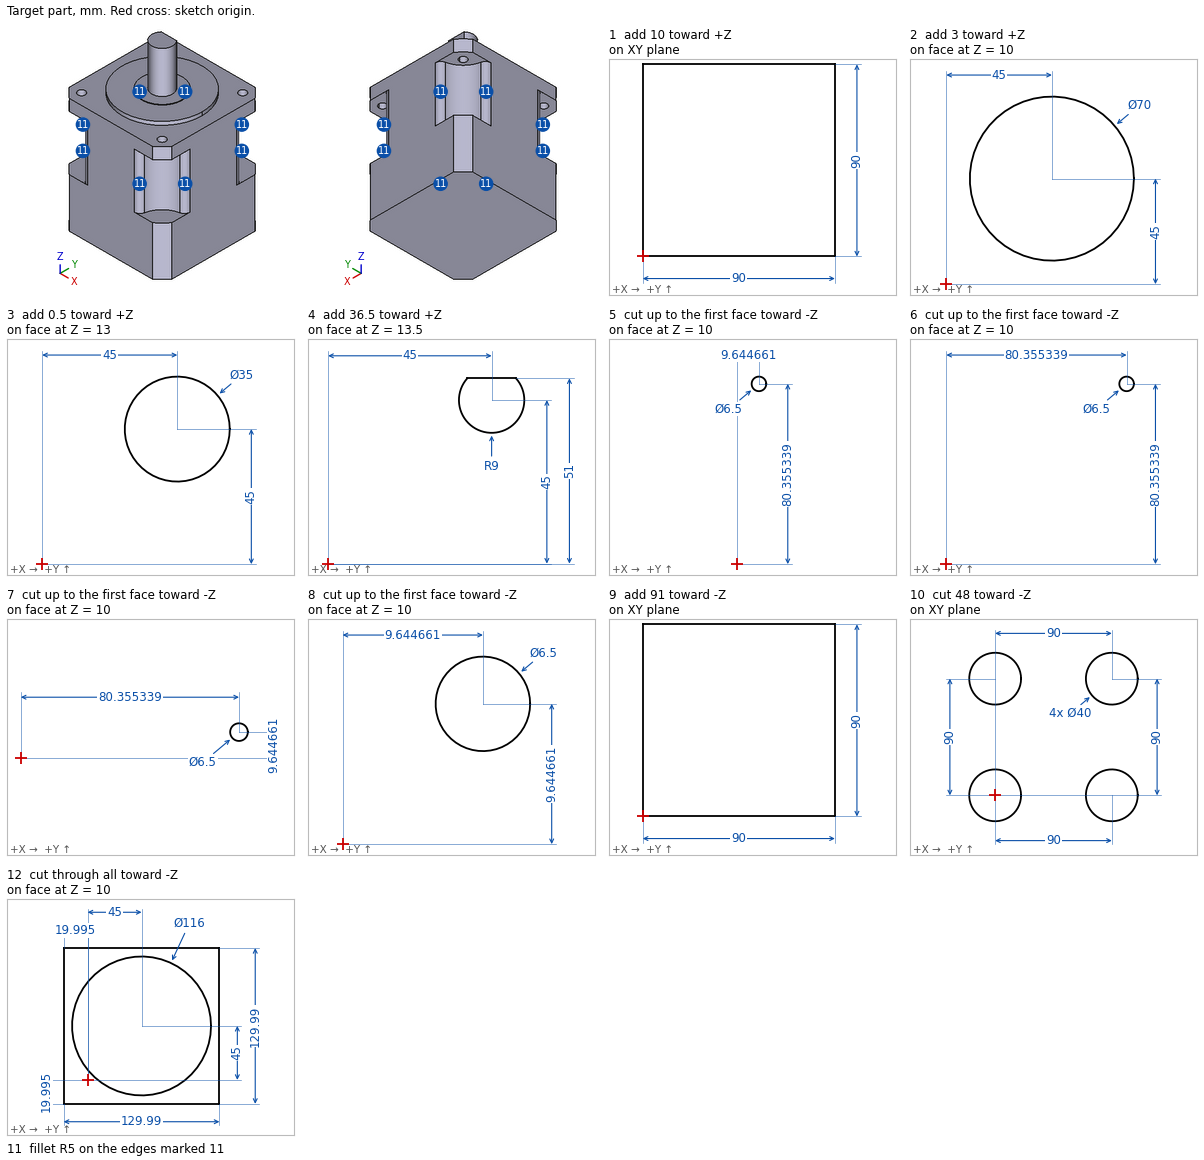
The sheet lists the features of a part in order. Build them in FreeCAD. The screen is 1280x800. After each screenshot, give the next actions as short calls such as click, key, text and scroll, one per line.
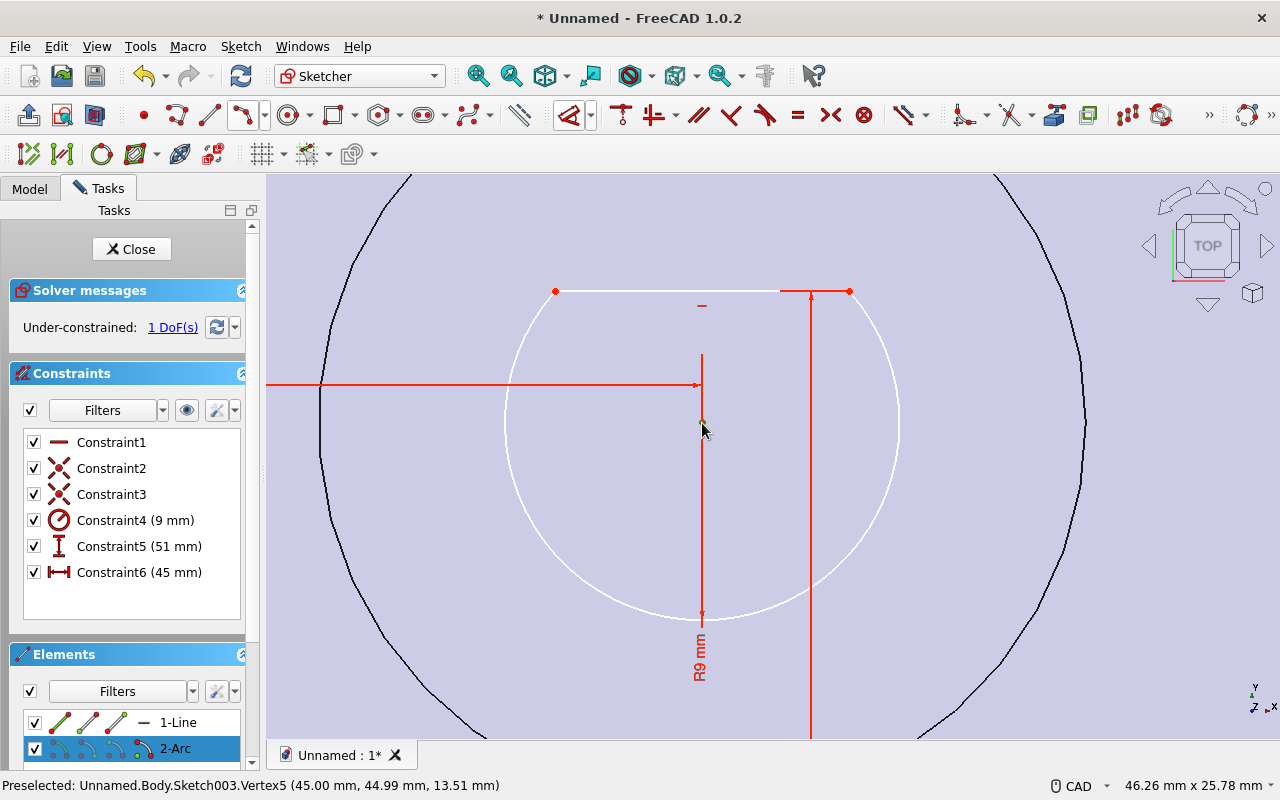
key(i)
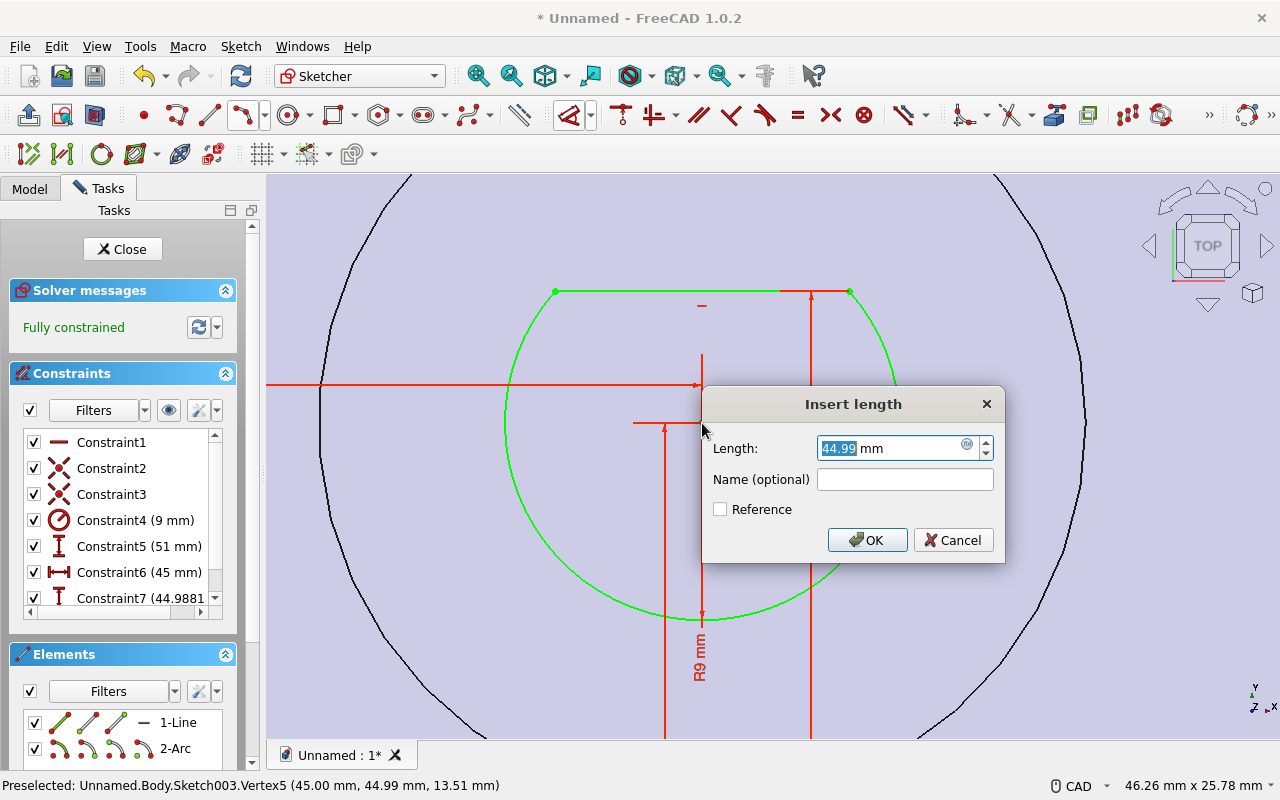
text(45)
key(Return)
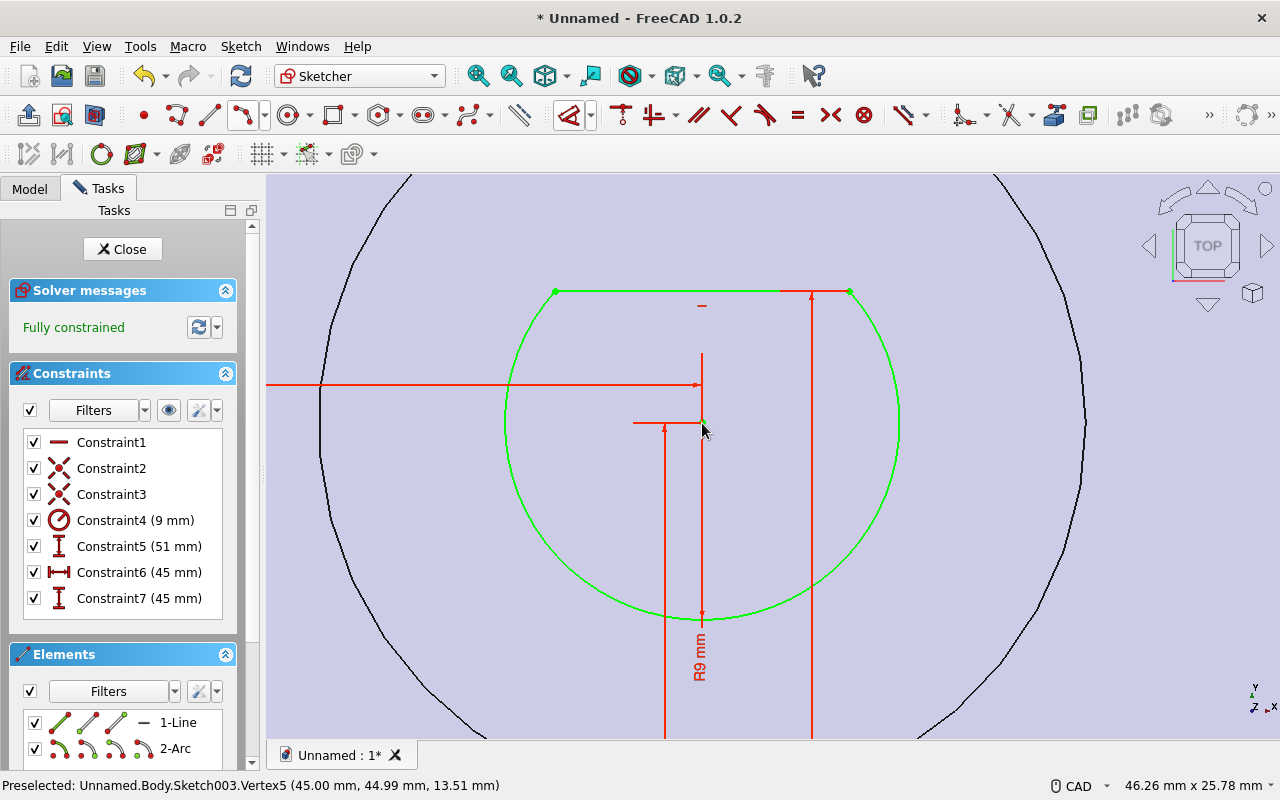
click(123, 249)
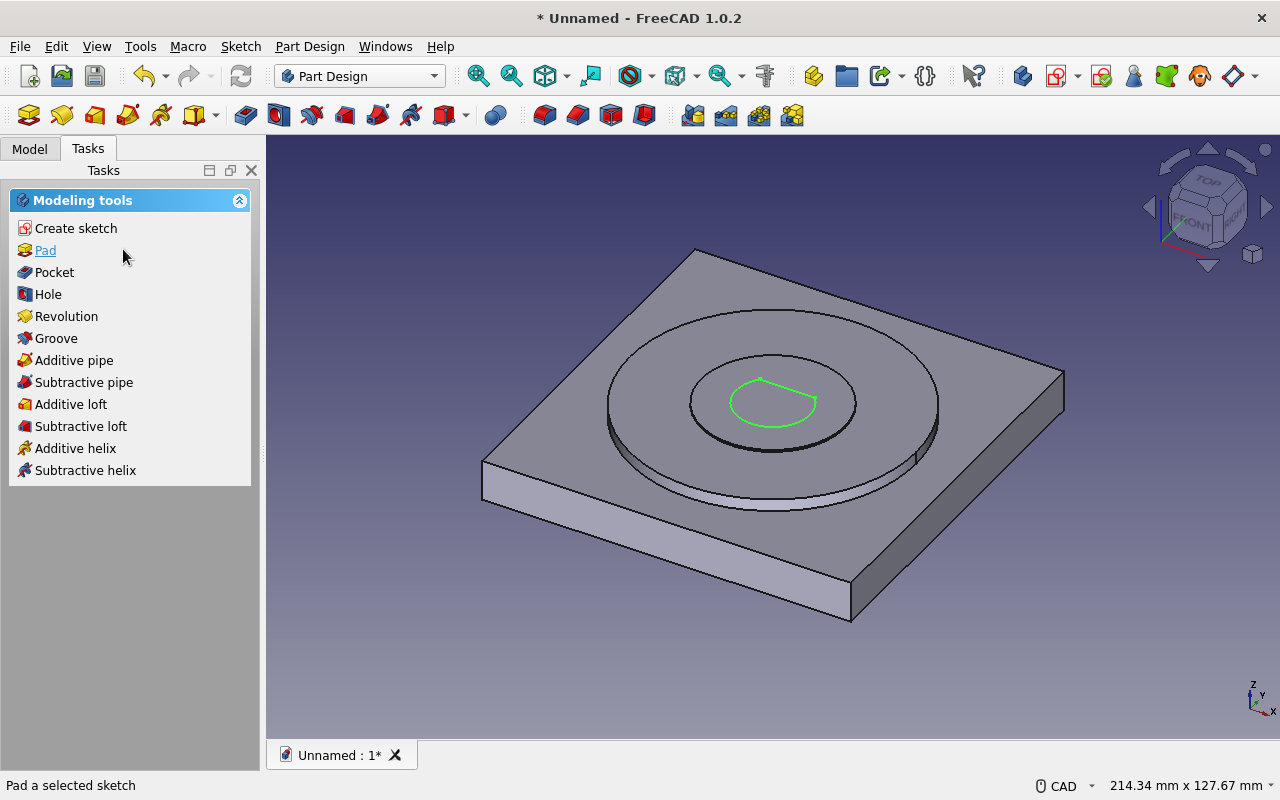
click(29, 116)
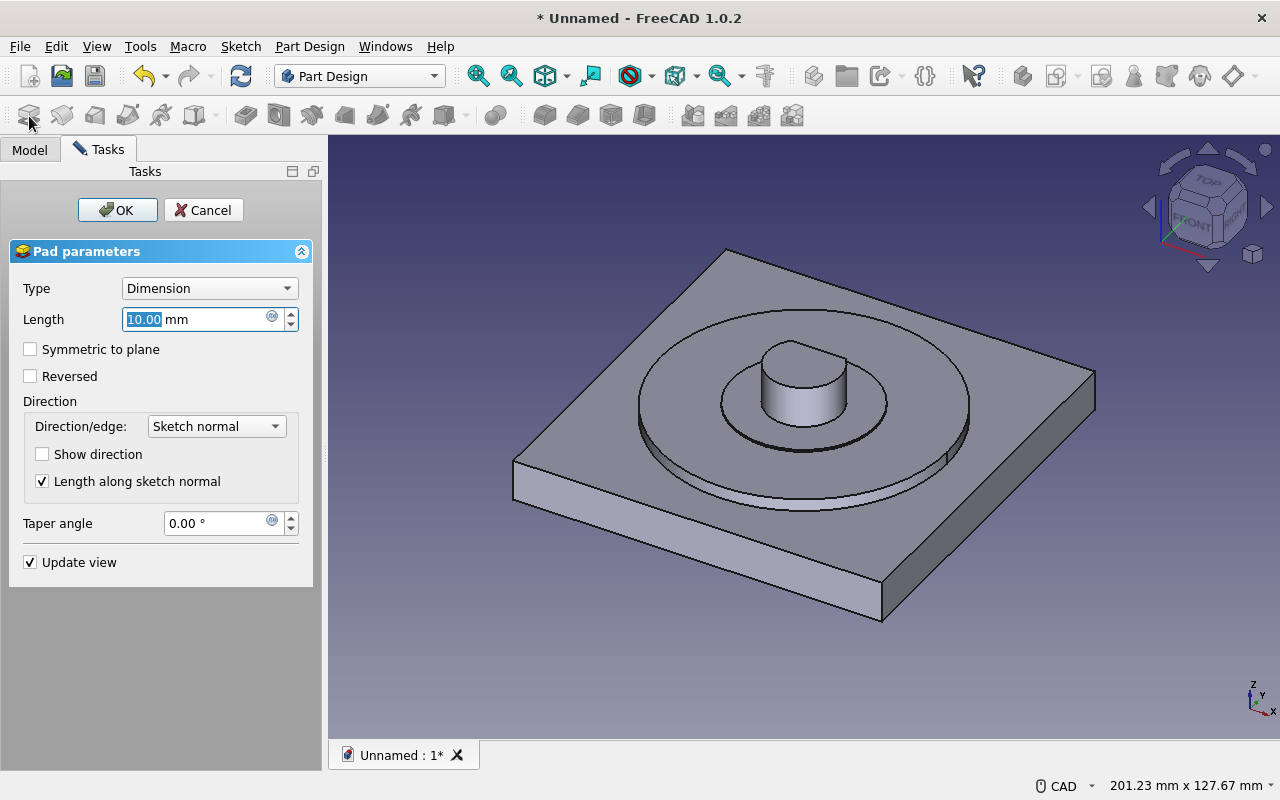
text(36.5)
key(Tab)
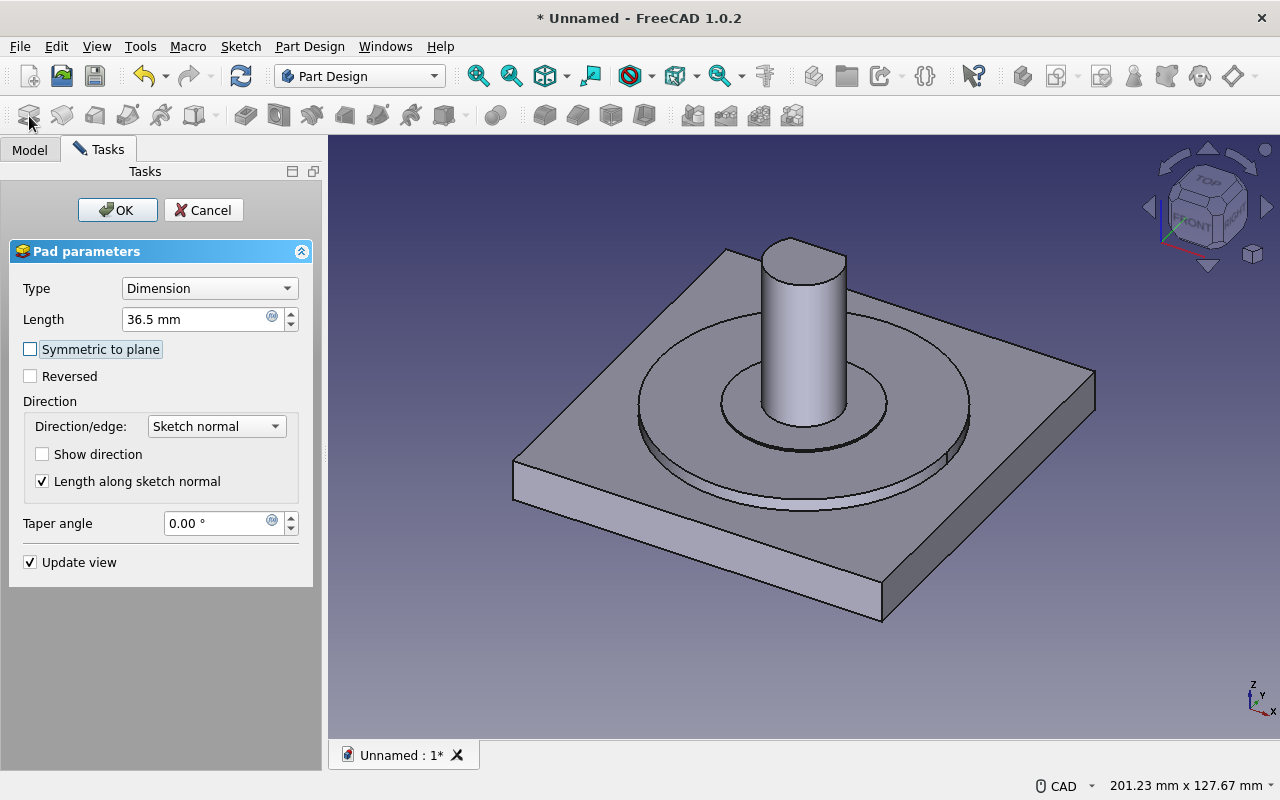
click(118, 210)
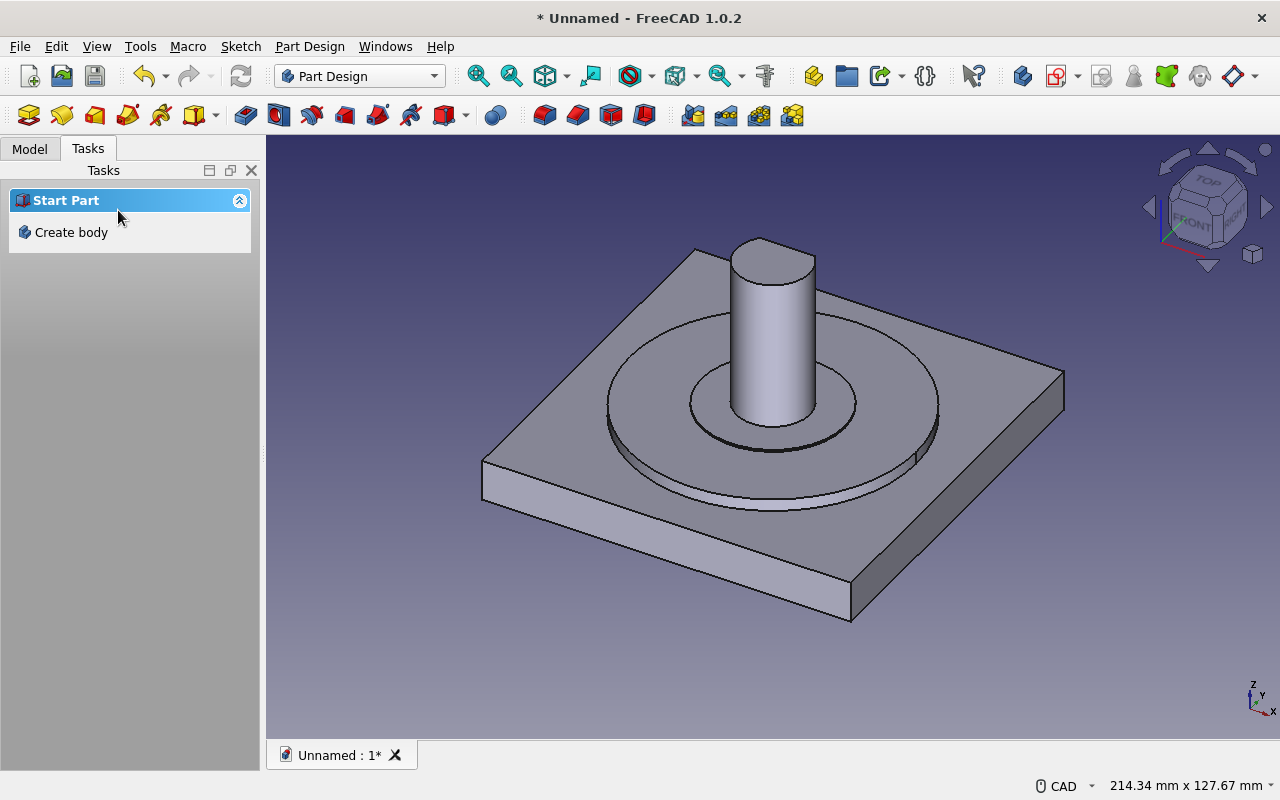
key(v)
key(f)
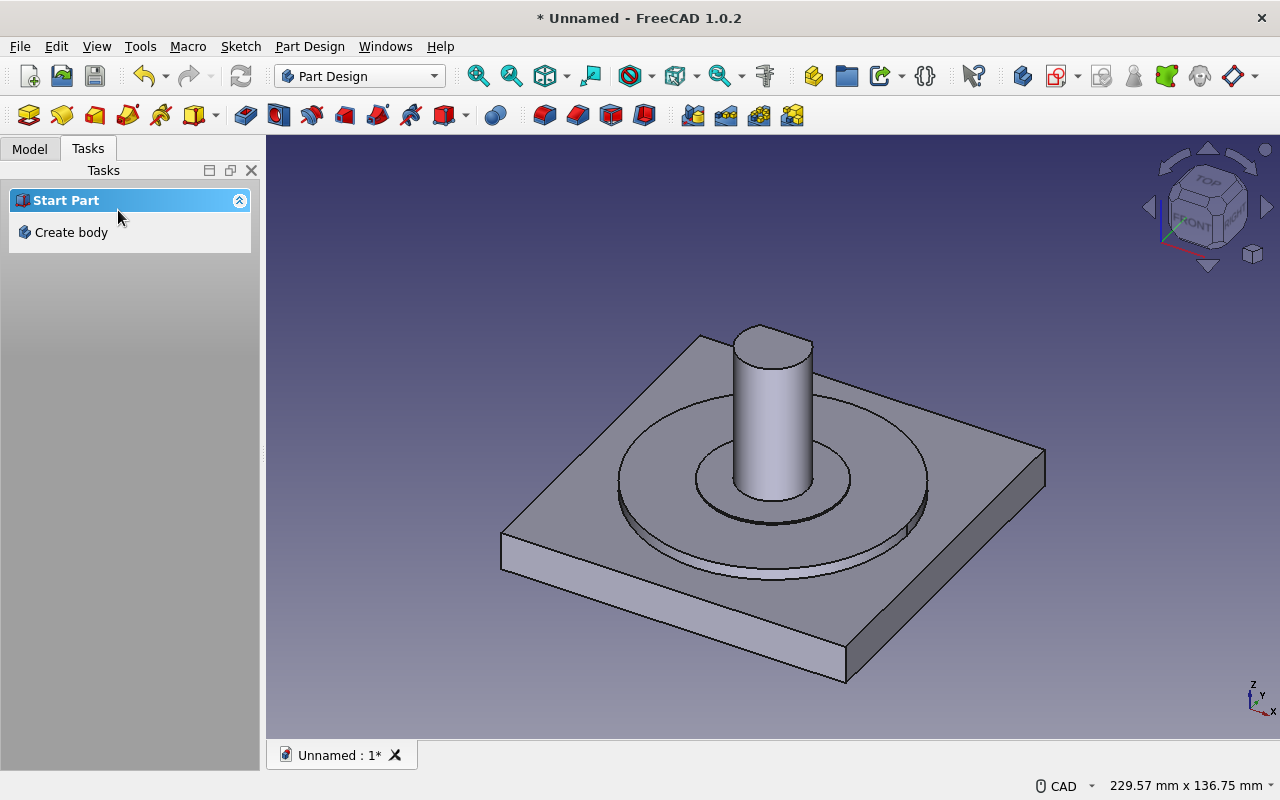
click(1006, 455)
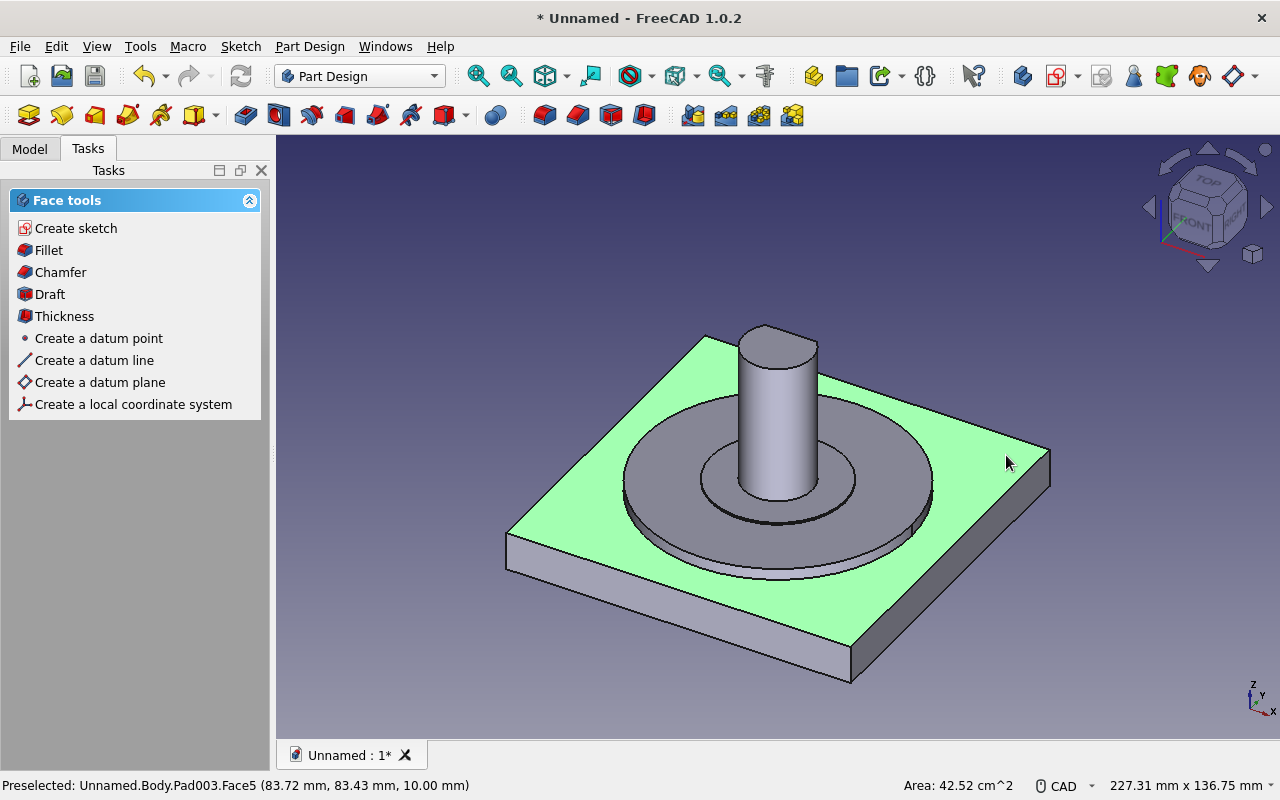
click(1056, 76)